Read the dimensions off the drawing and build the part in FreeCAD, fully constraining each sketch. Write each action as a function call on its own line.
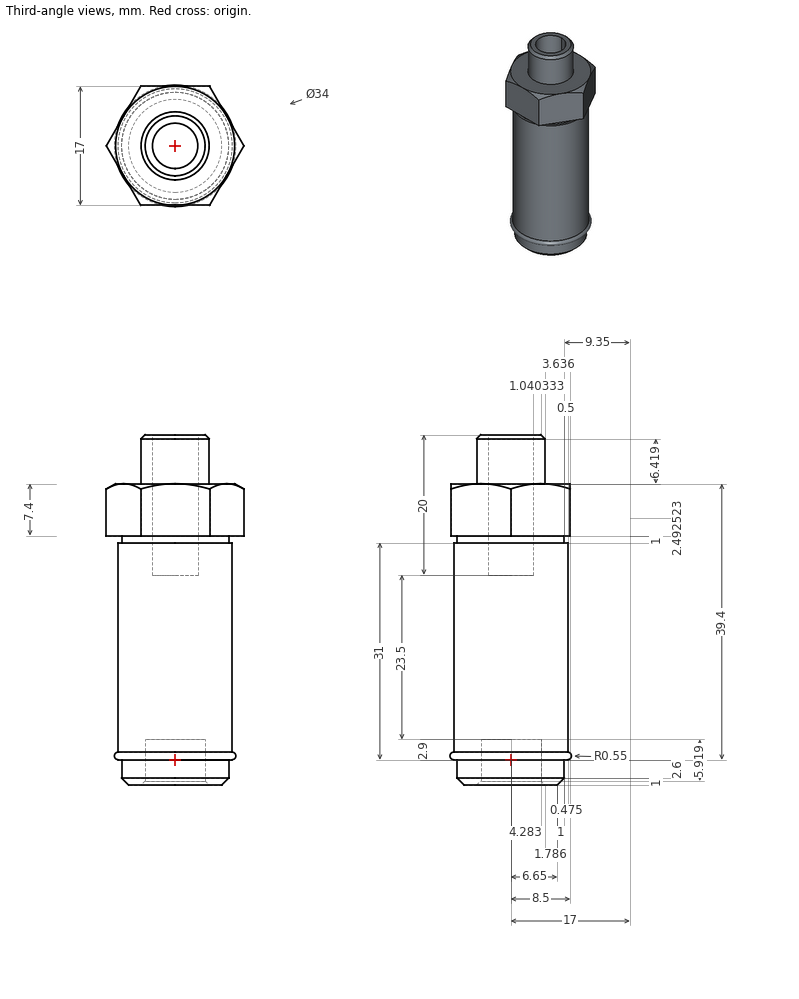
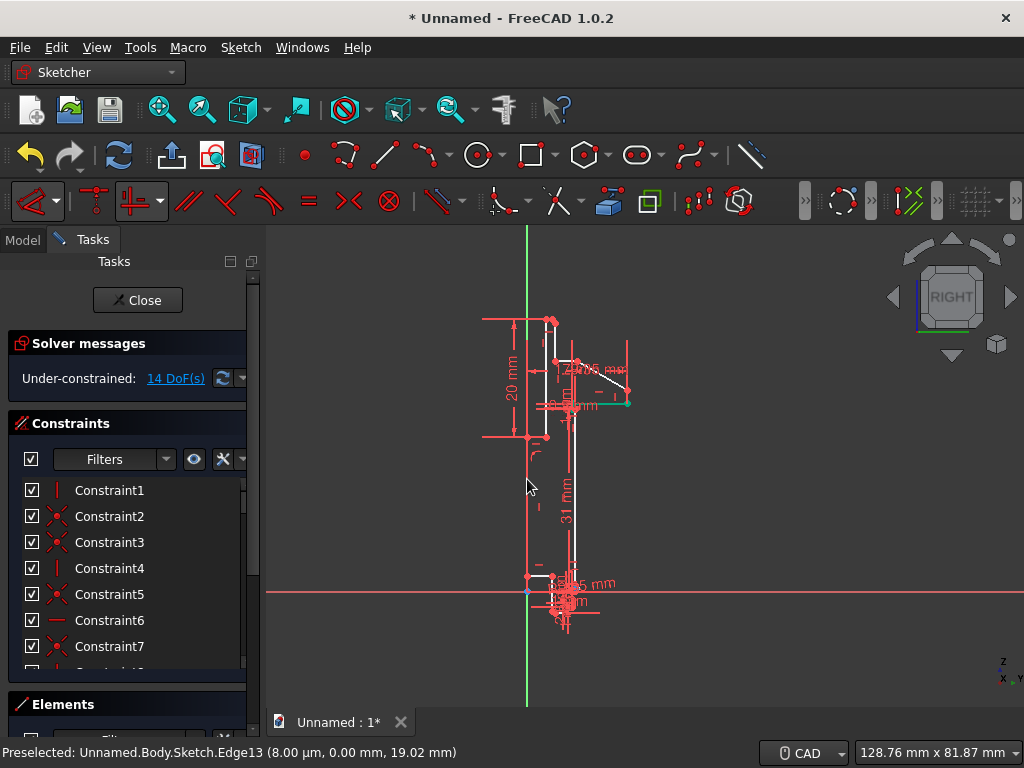
key(i)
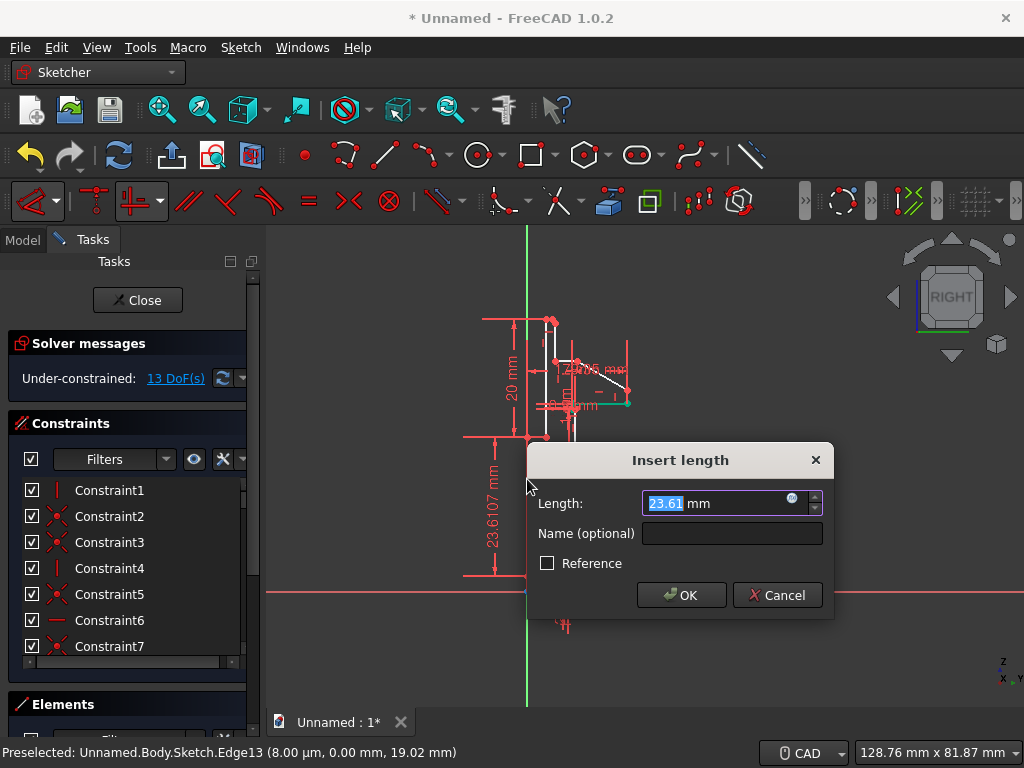
text(23.5)
key(Return)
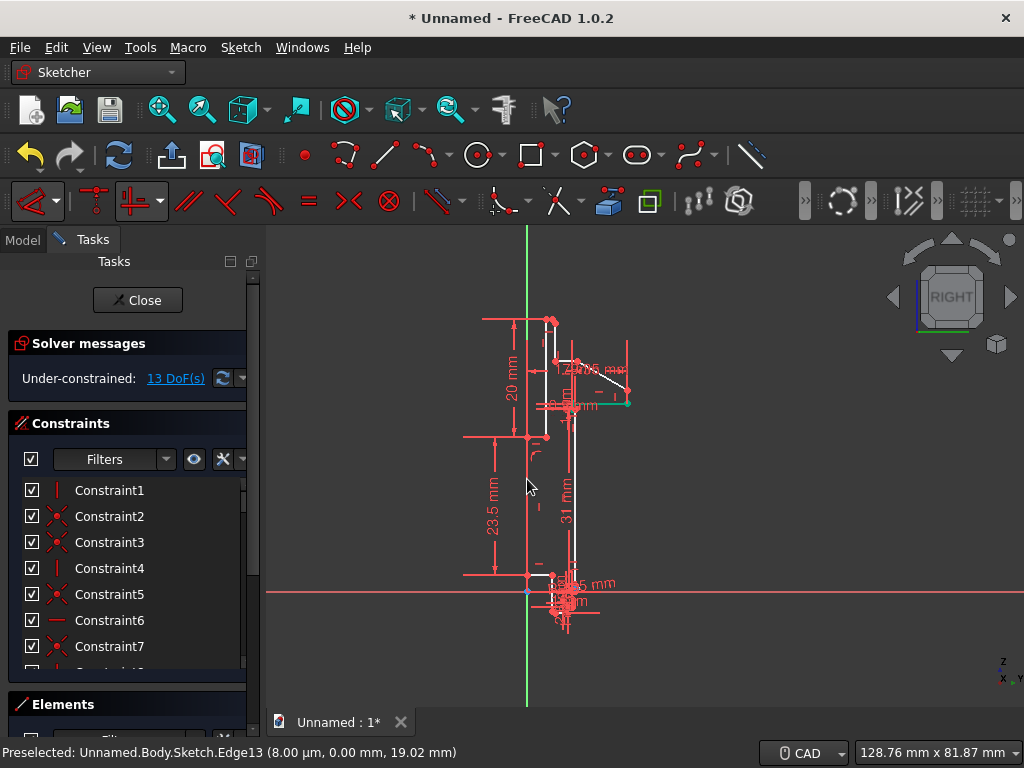
click(577, 361)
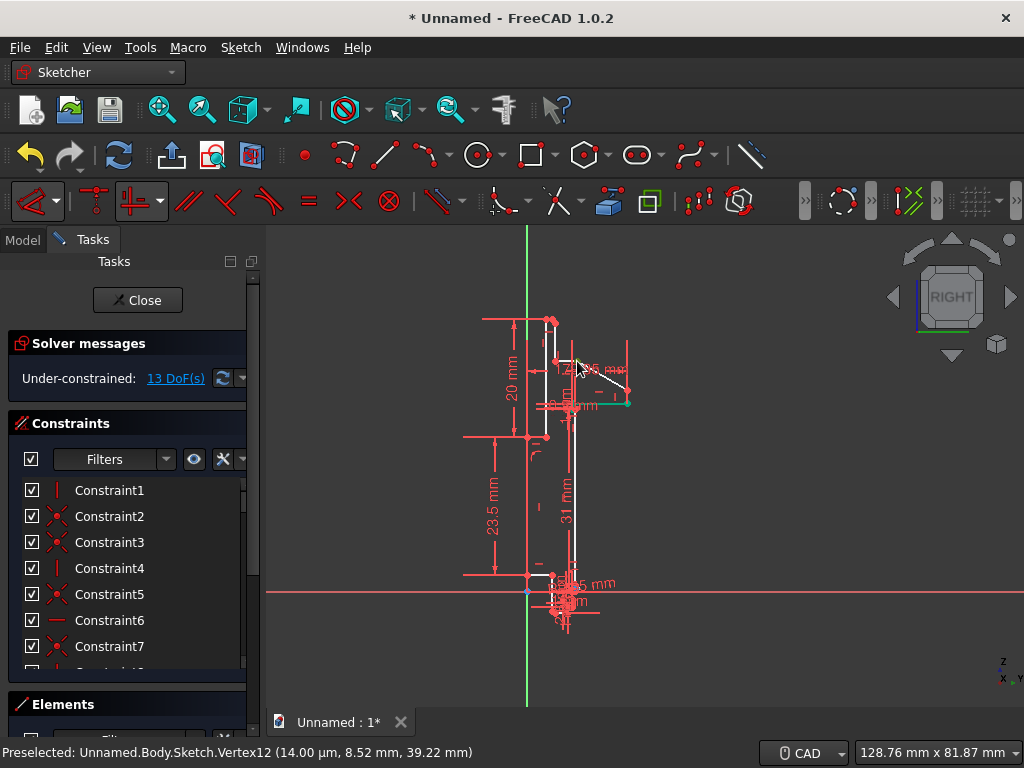
key(l)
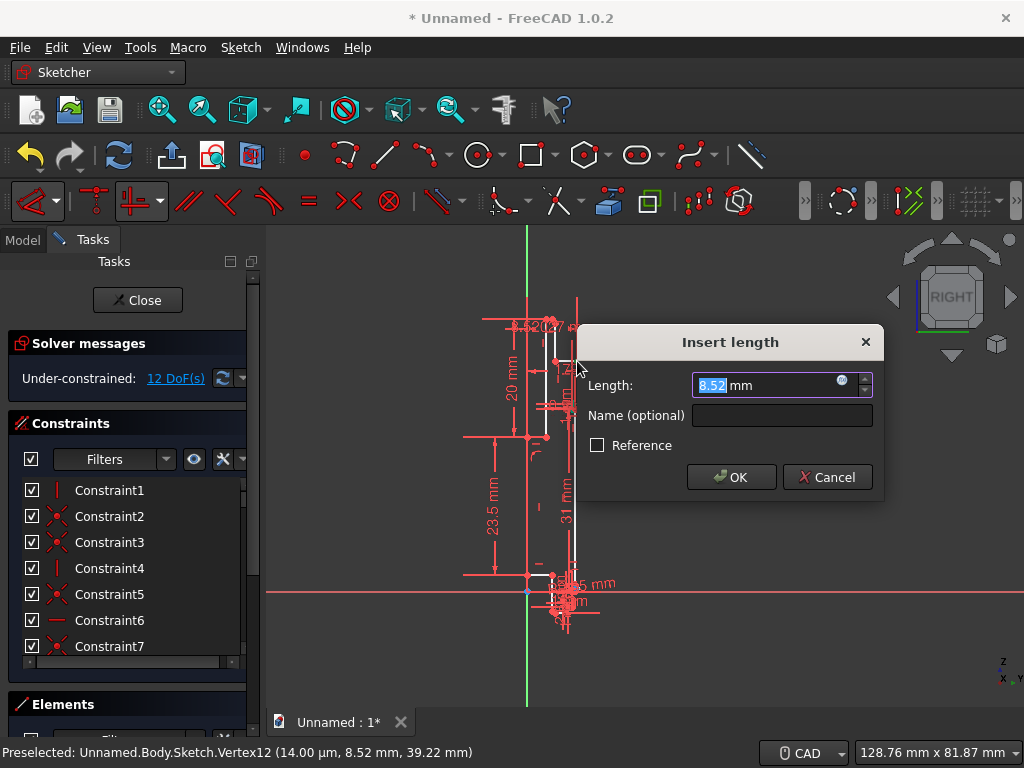
text(8.5)
key(Return)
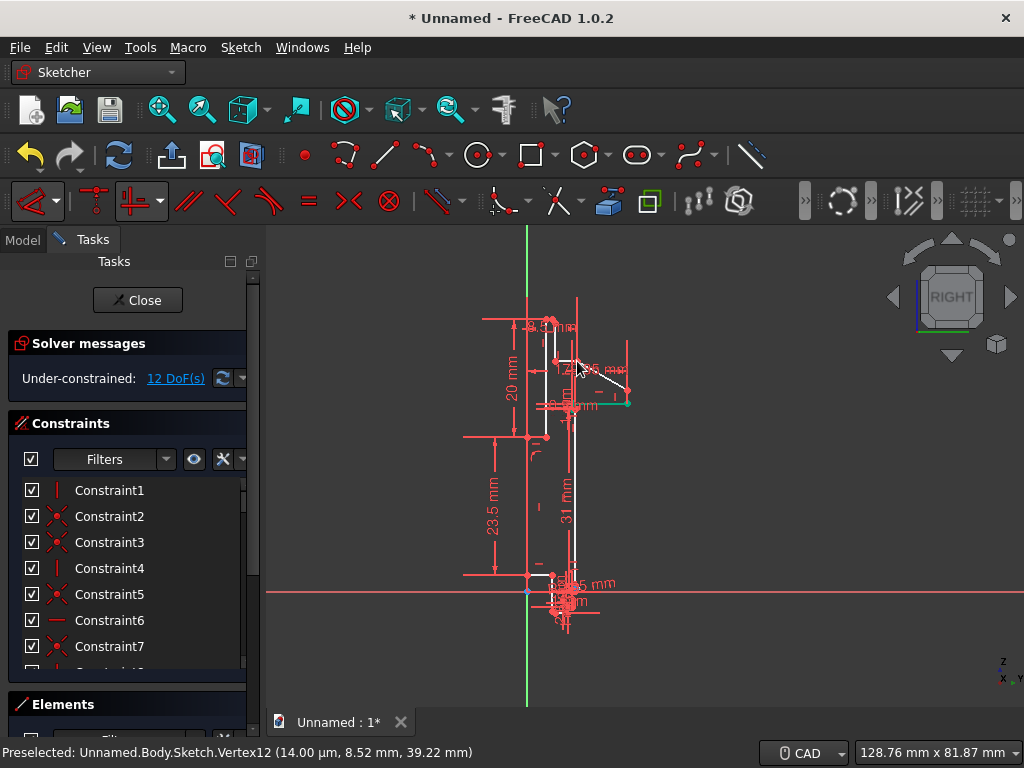
scroll(527, 575, up, 5)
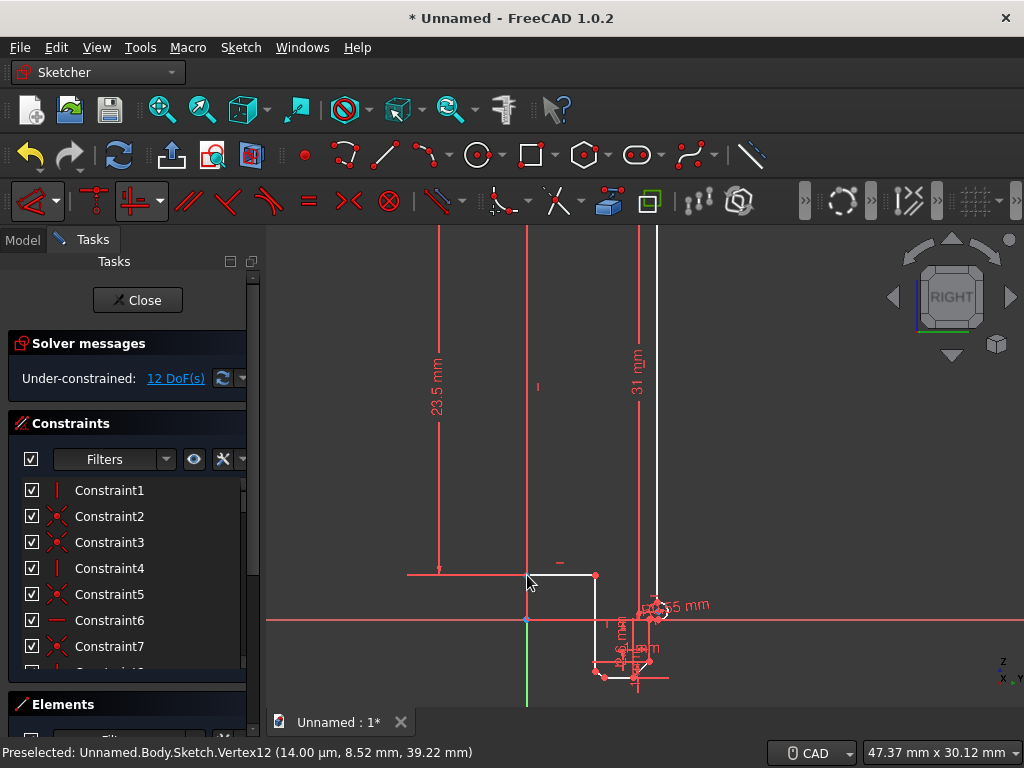
click(527, 575)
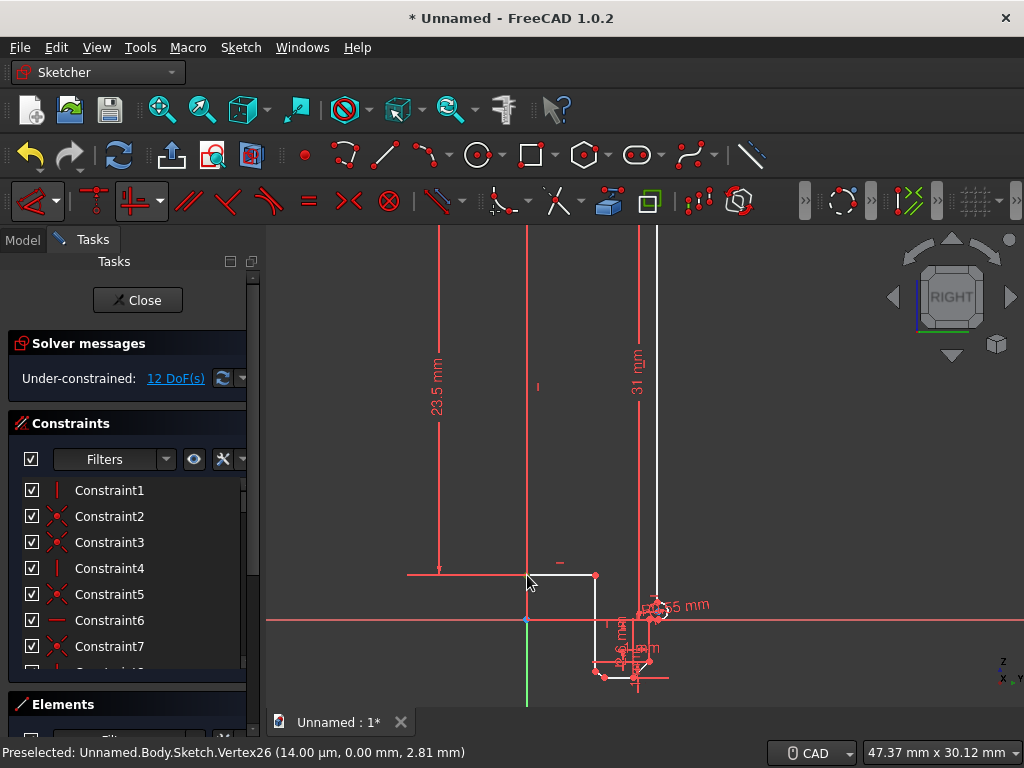
key(i)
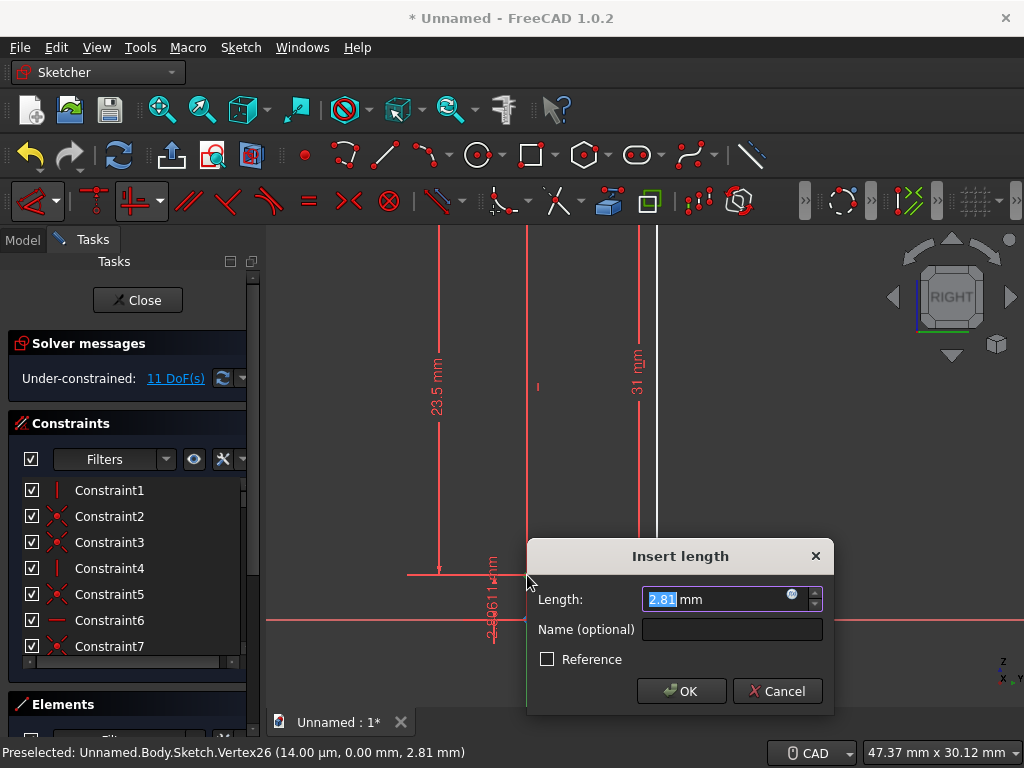
text(2.9)
key(Return)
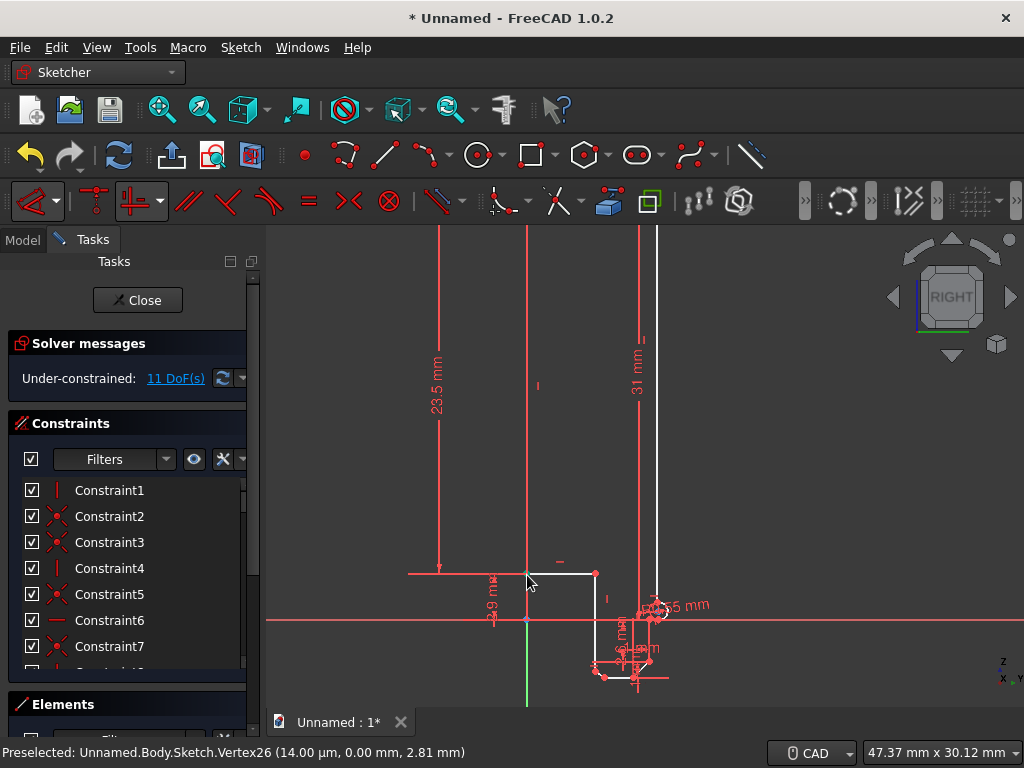
scroll(526, 576, down, 5)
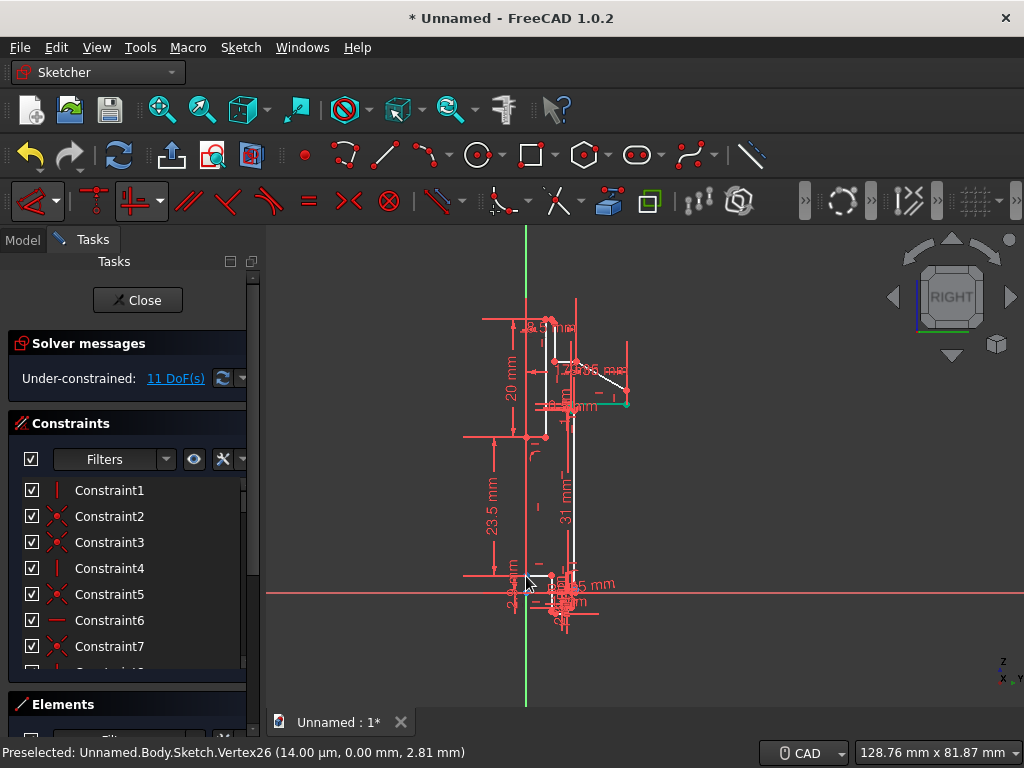
scroll(570, 362, up, 4)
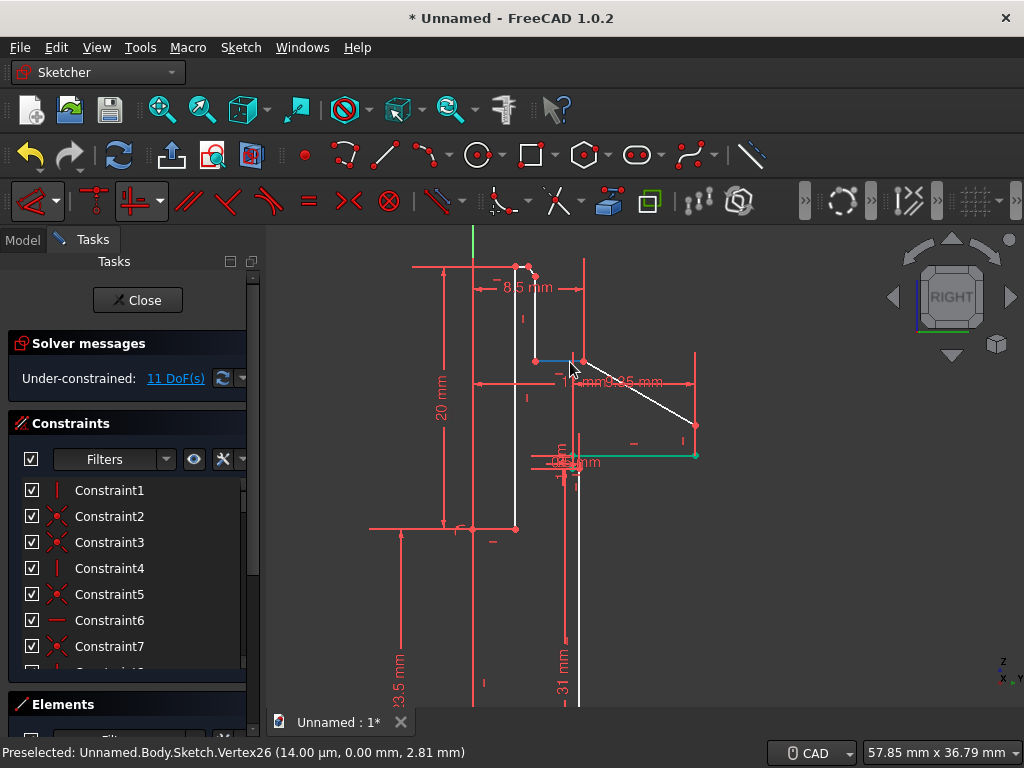
click(569, 361)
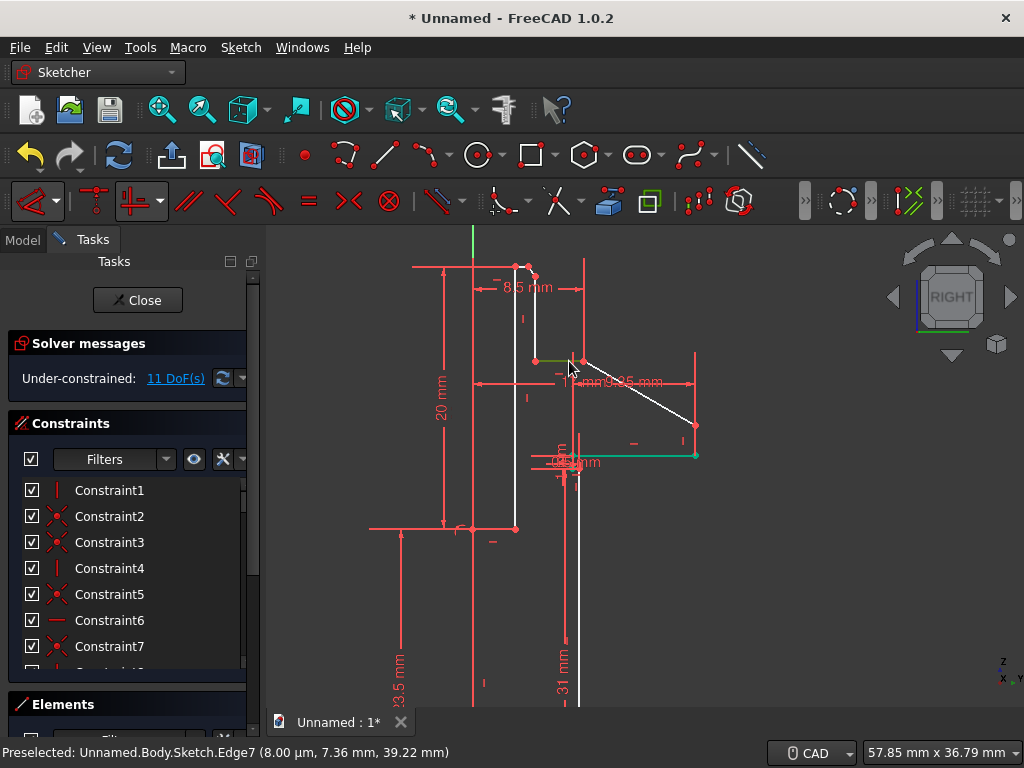
key(l)